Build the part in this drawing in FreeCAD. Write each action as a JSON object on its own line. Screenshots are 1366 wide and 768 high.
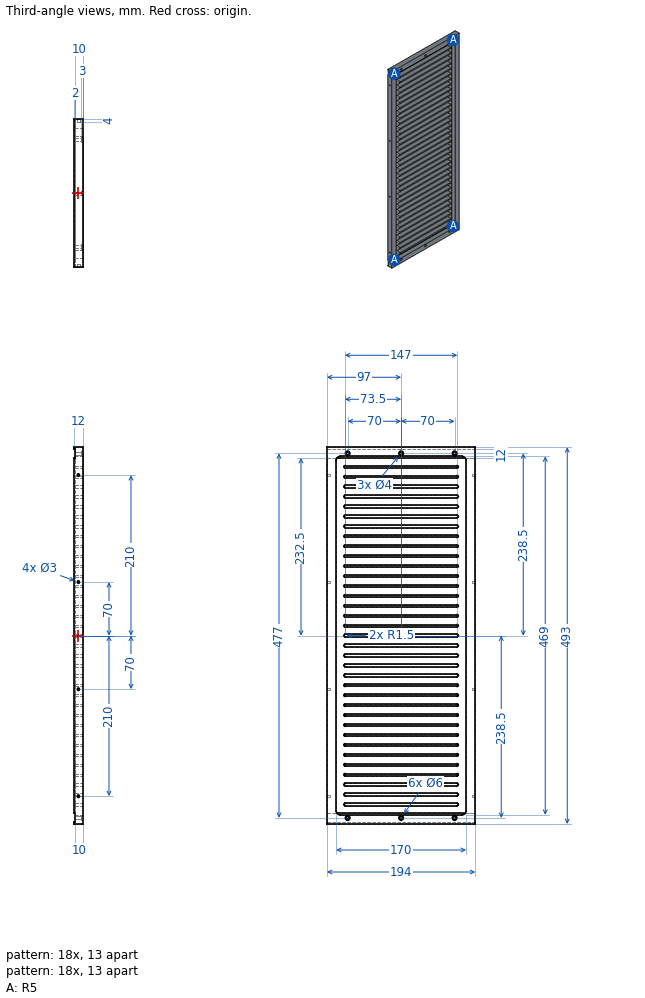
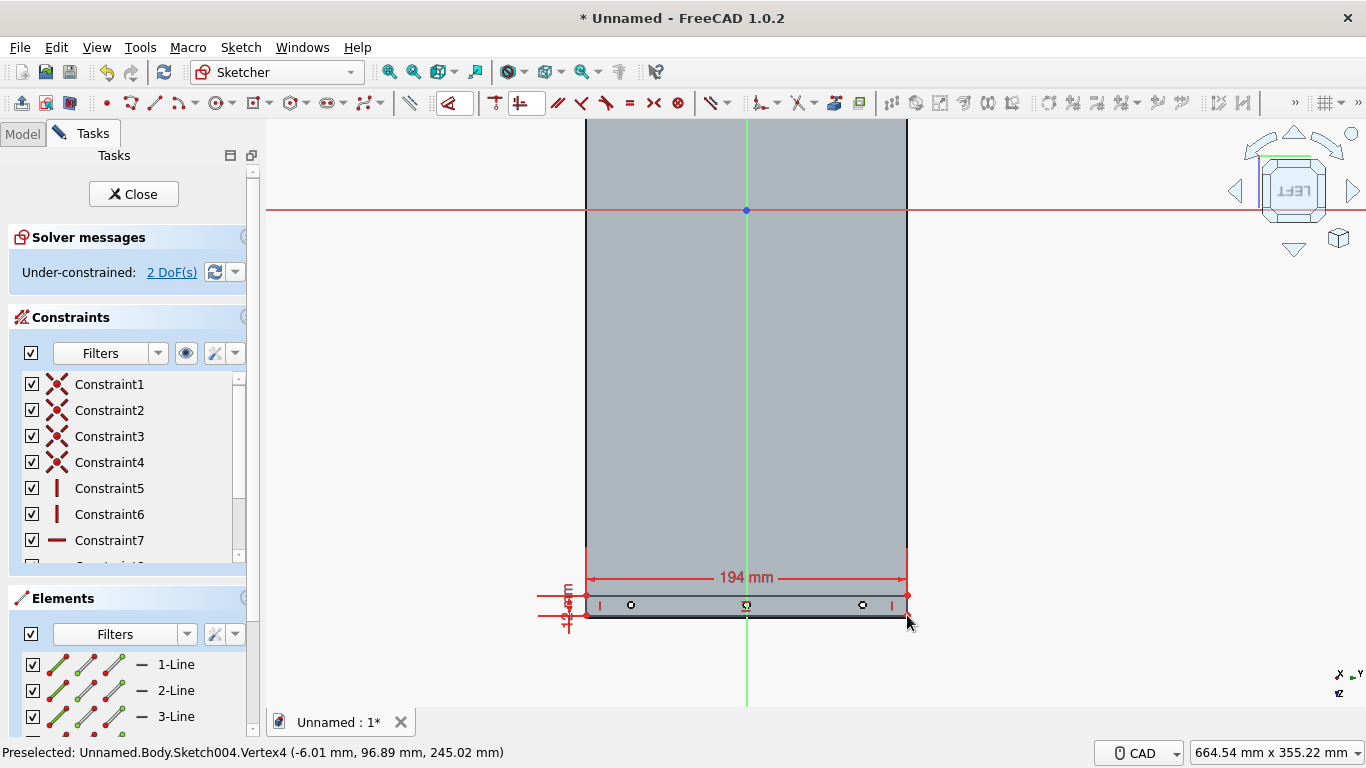
{"action": "left_click", "coordinate": [586, 596]}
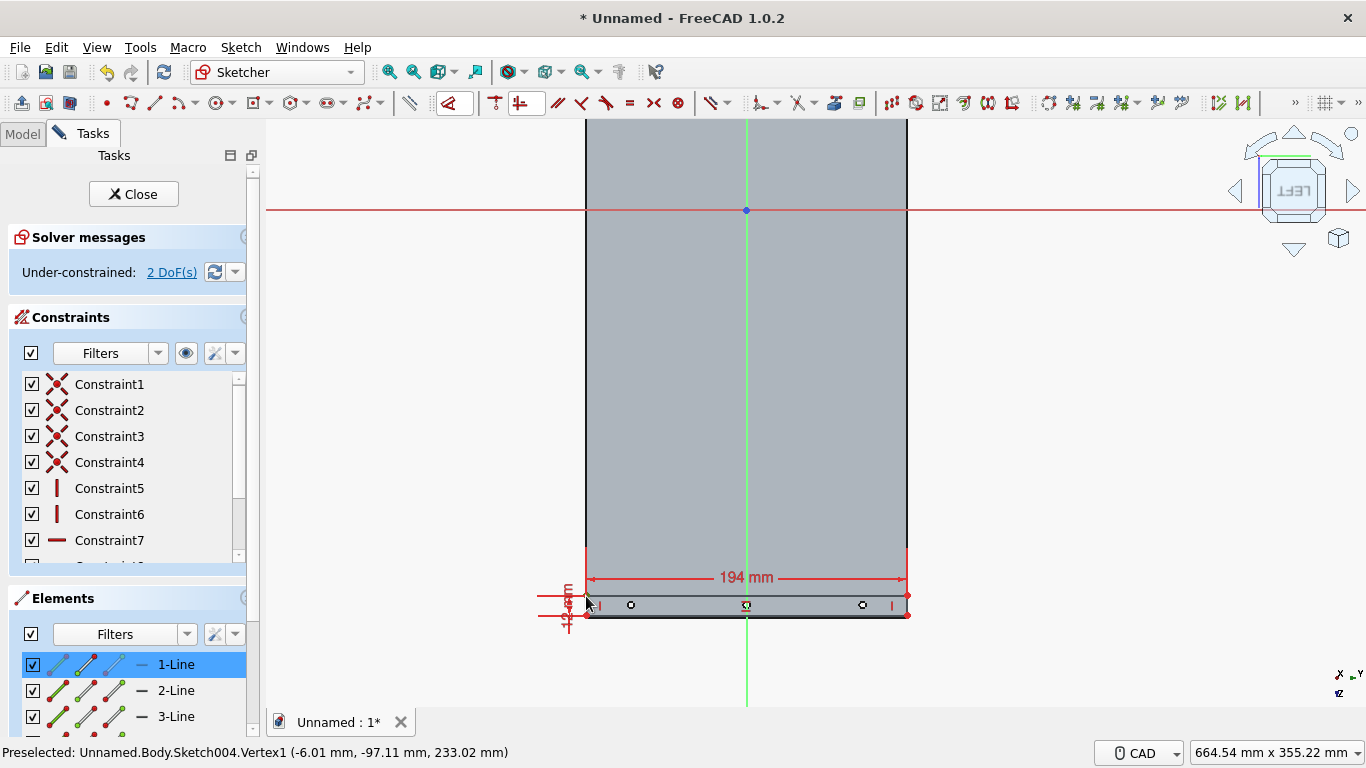
{"action": "left_click", "coordinate": [468, 104]}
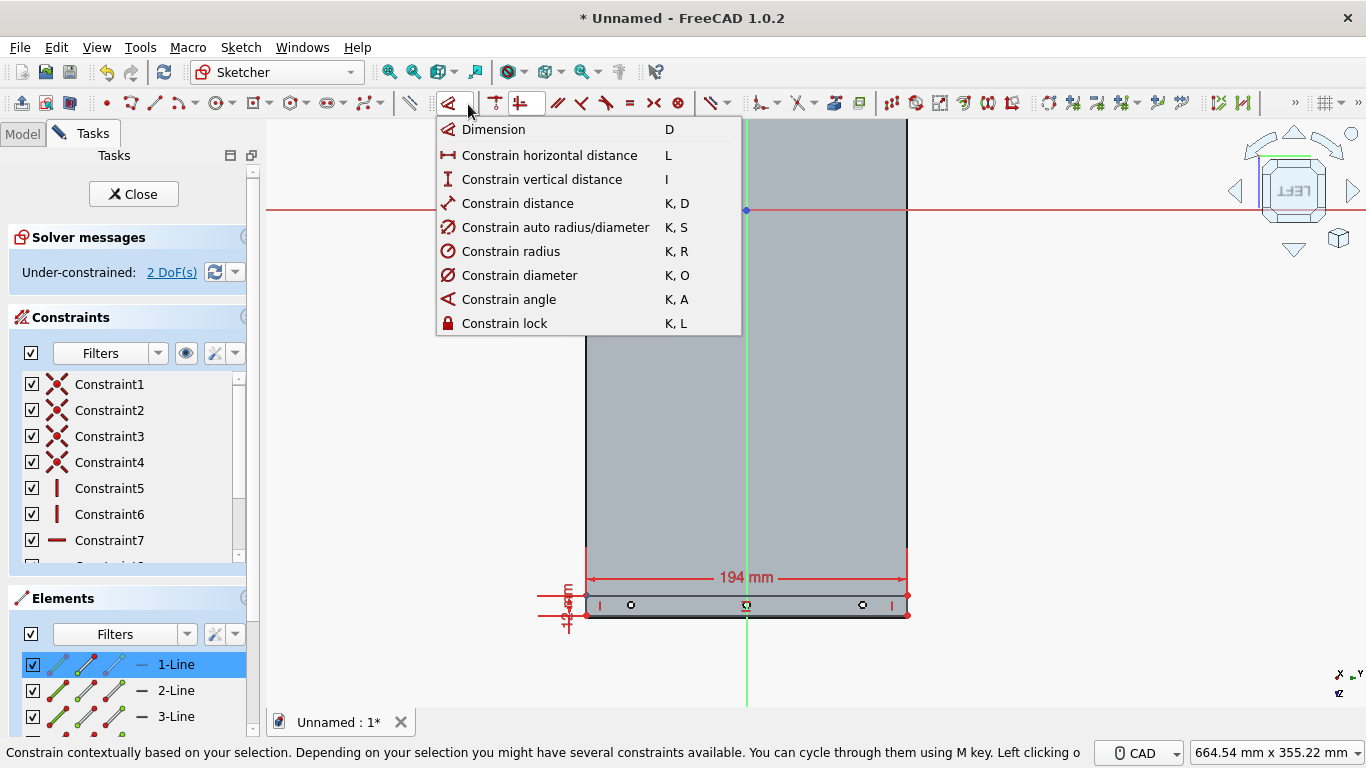
{"action": "left_click", "coordinate": [589, 155]}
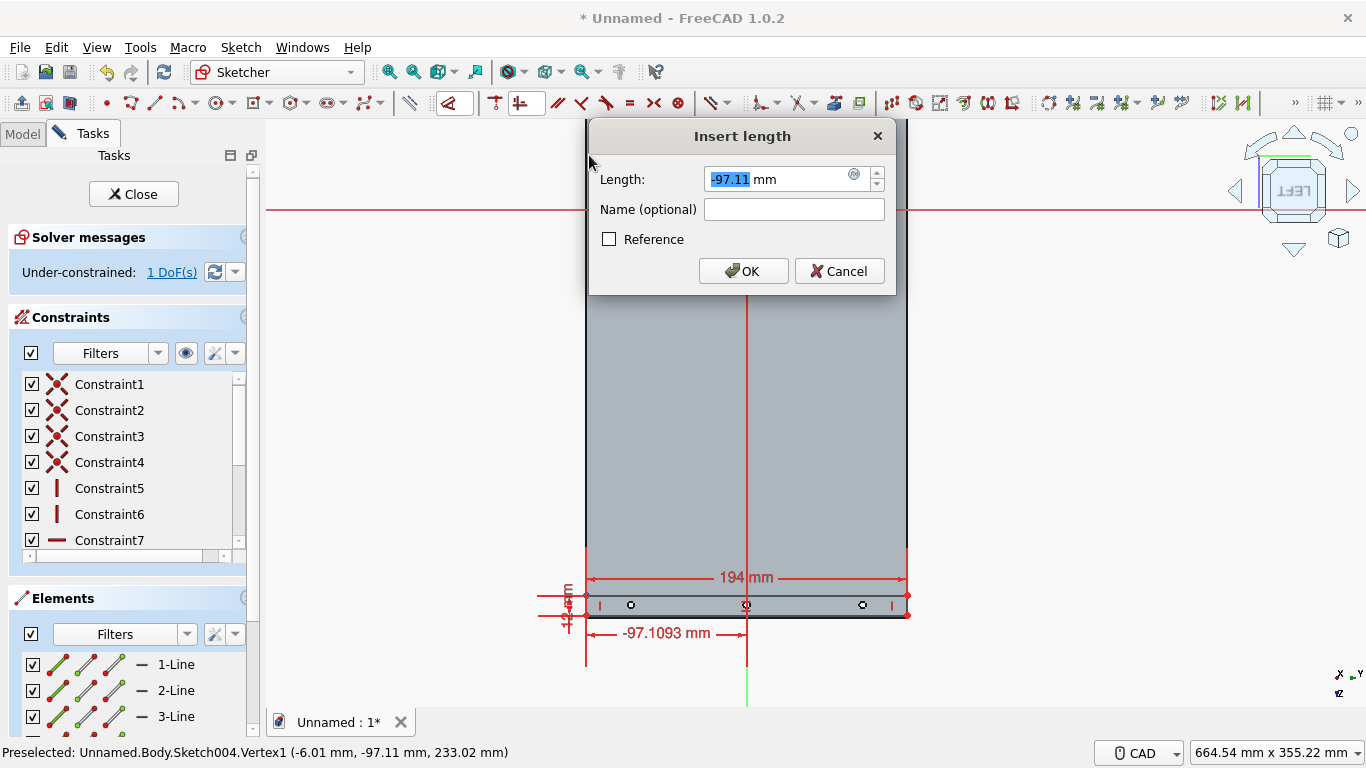
{"action": "type", "text": "-97"}
{"action": "key", "text": "Return"}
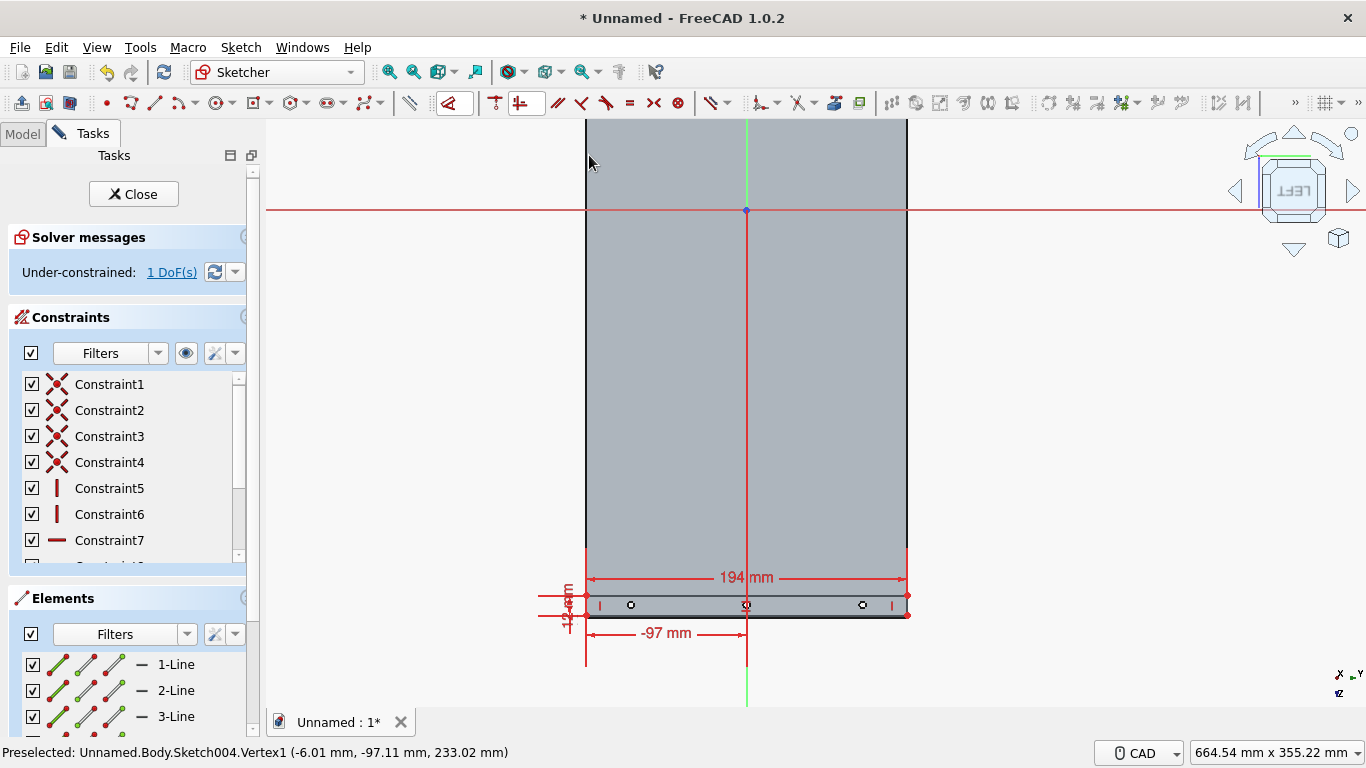
{"action": "left_click", "coordinate": [586, 596]}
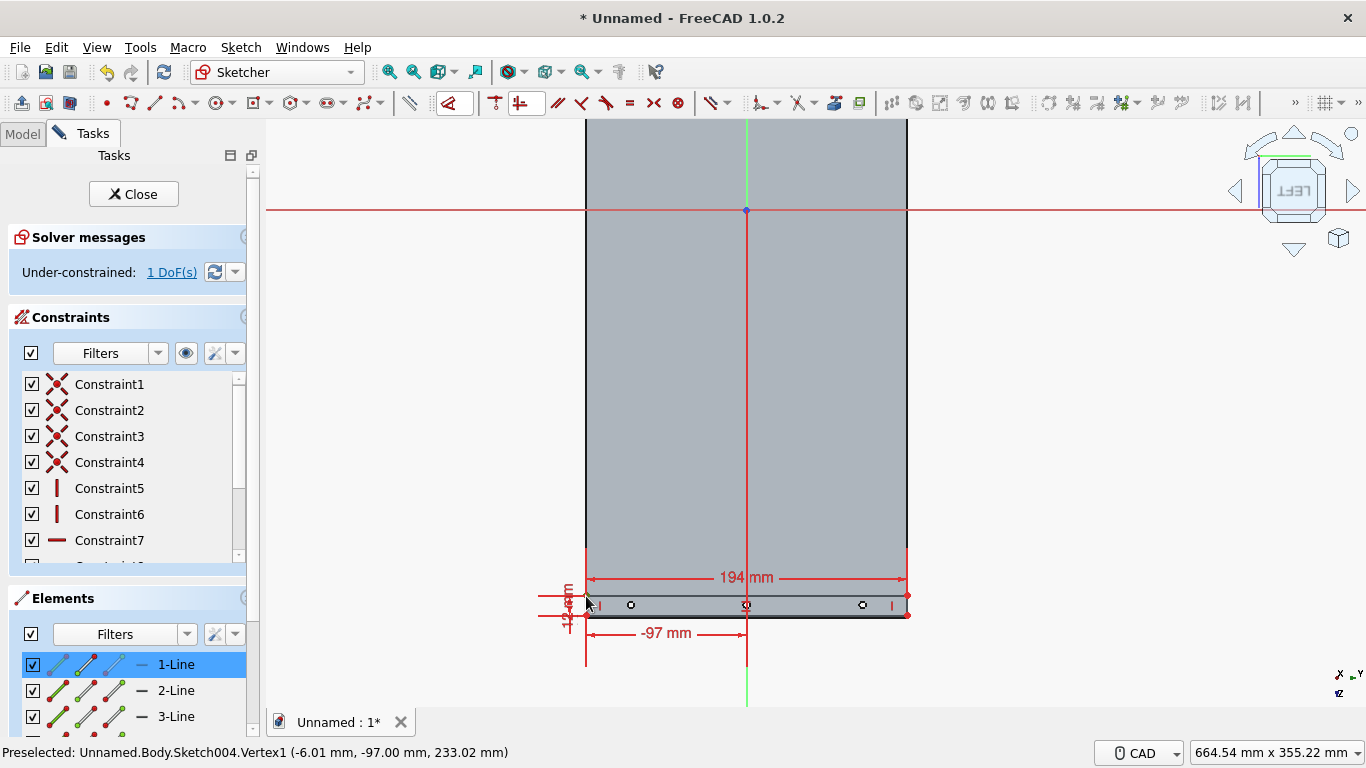
{"action": "left_click", "coordinate": [468, 104]}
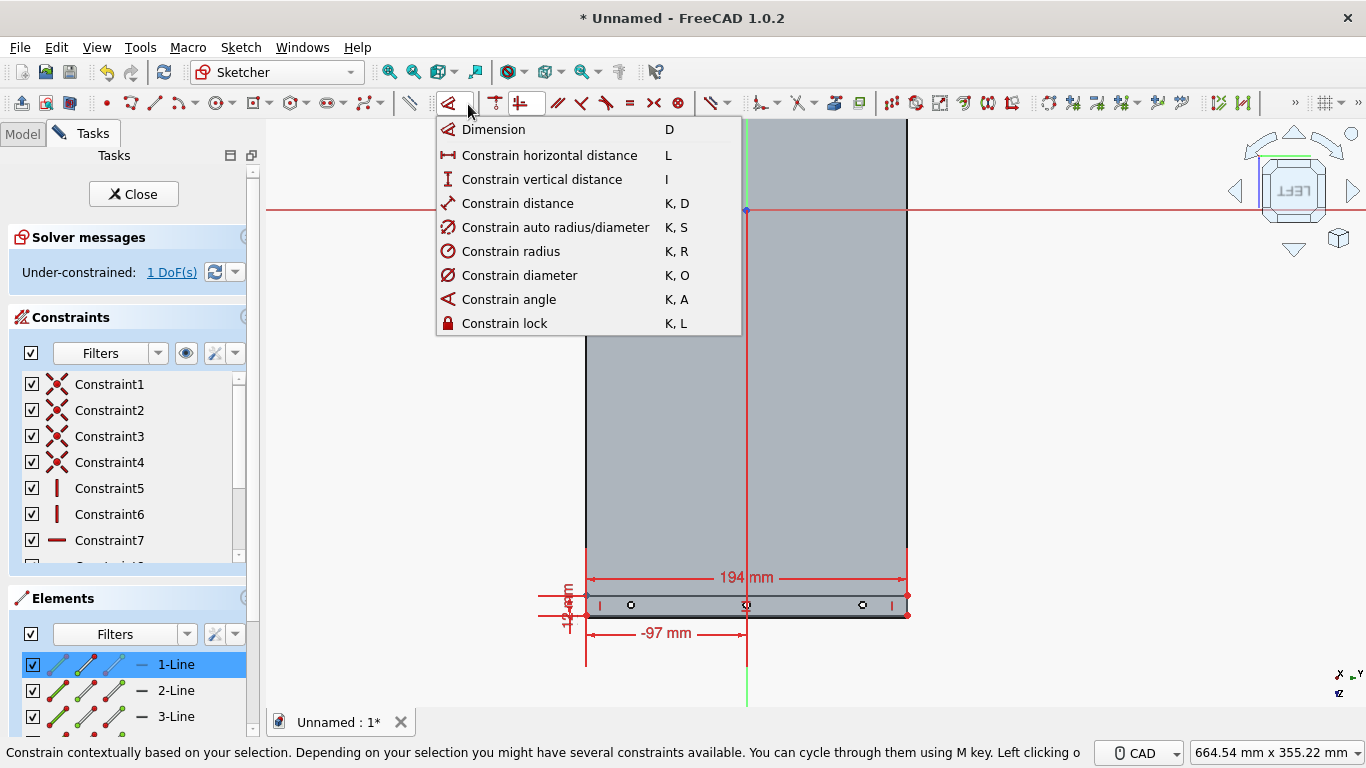
{"action": "left_click", "coordinate": [589, 179]}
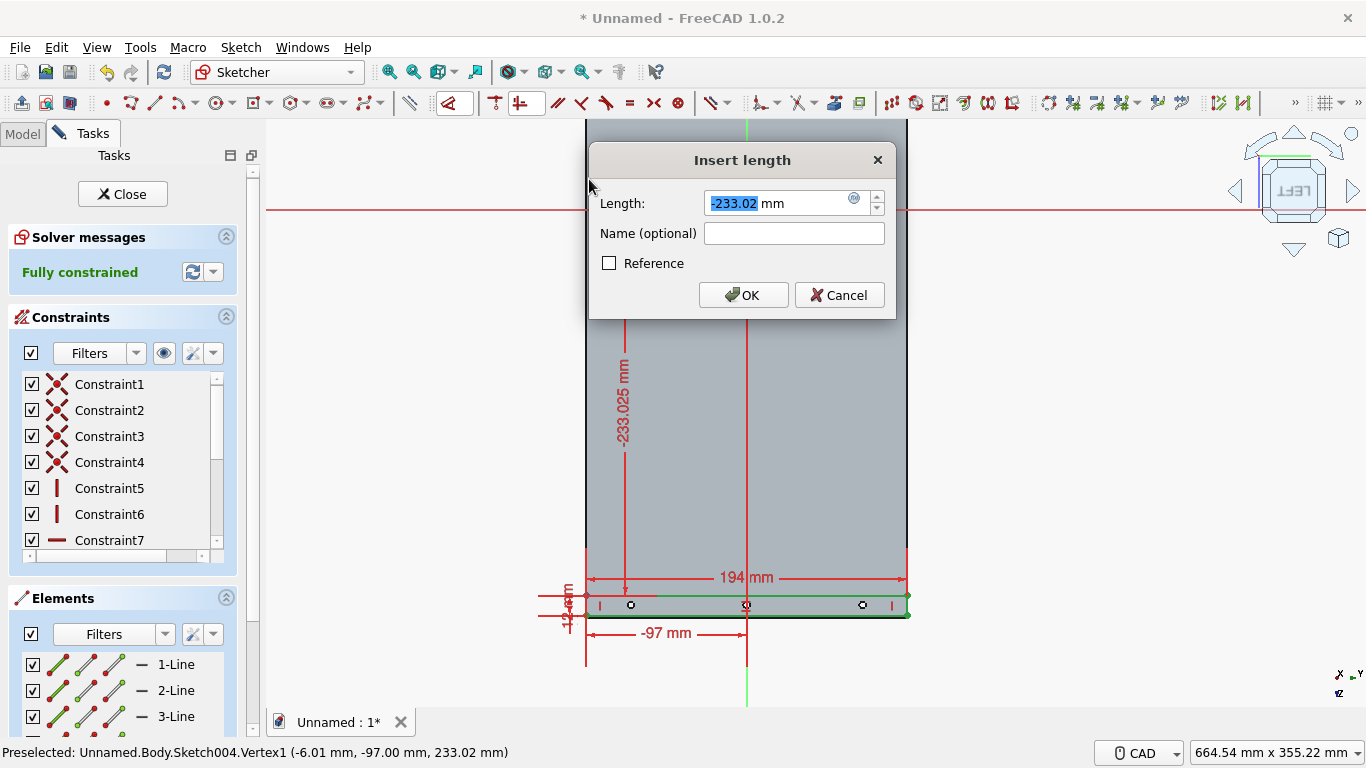
{"action": "type", "text": "-232.5"}
{"action": "key", "text": "Return"}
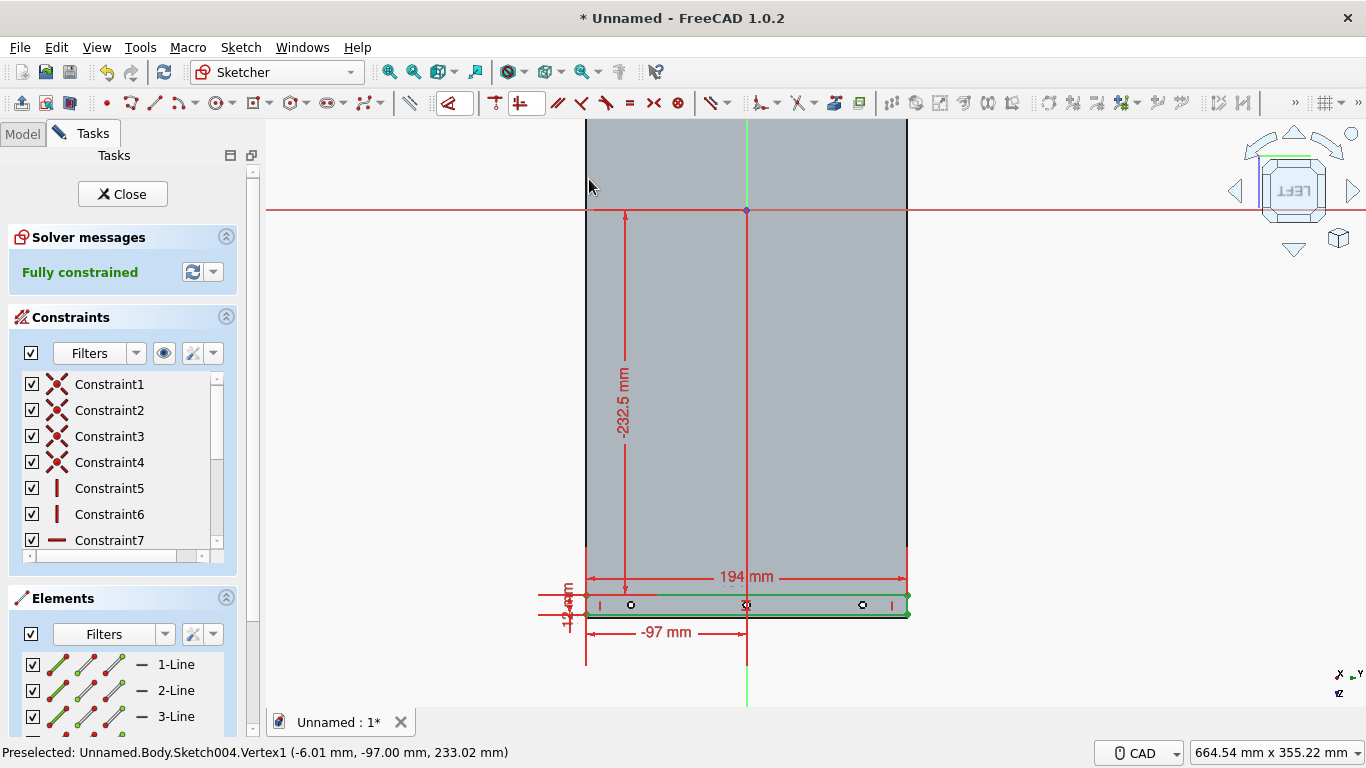
{"action": "left_click", "coordinate": [123, 194]}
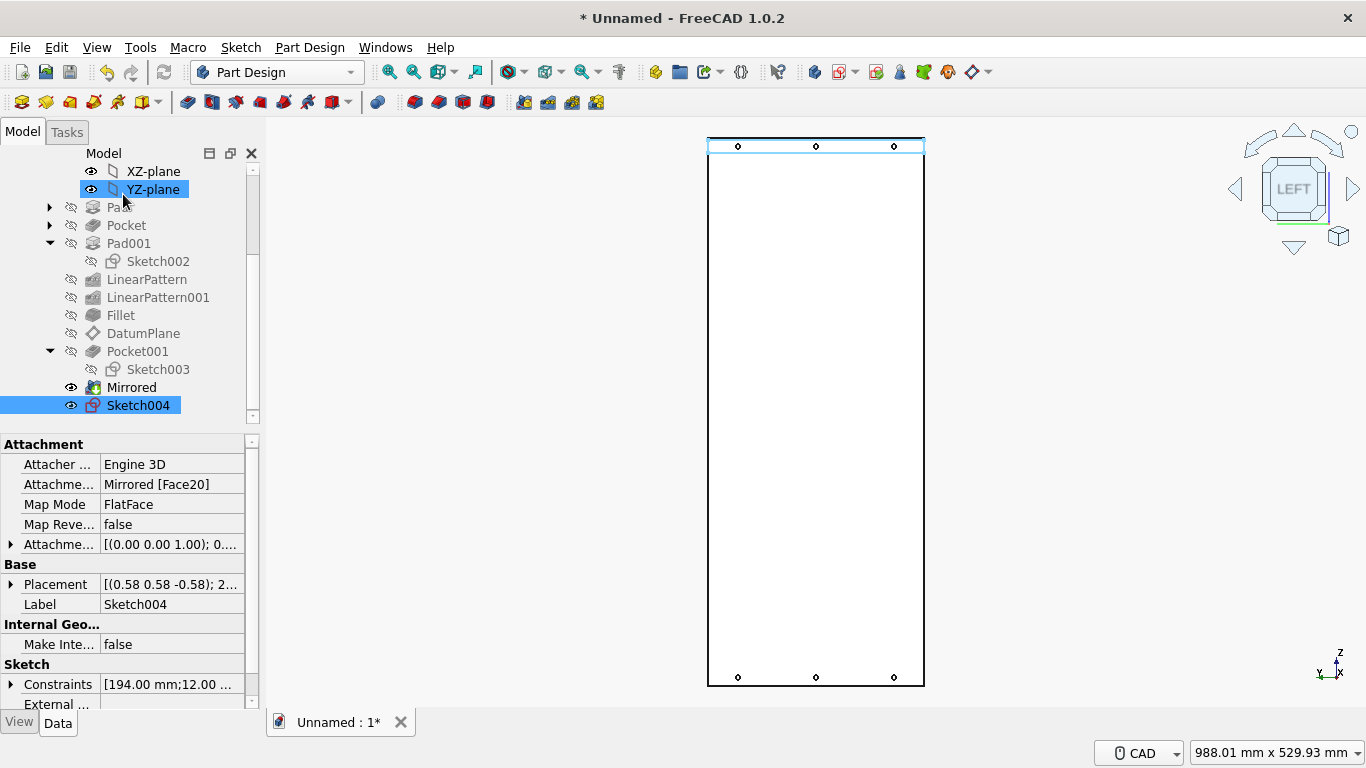
{"action": "left_click", "coordinate": [188, 102]}